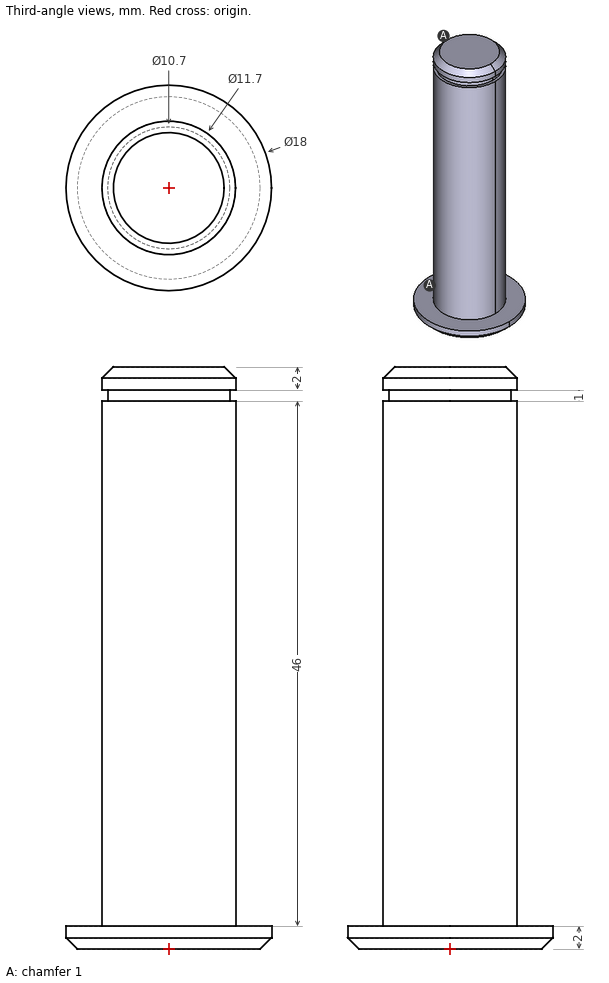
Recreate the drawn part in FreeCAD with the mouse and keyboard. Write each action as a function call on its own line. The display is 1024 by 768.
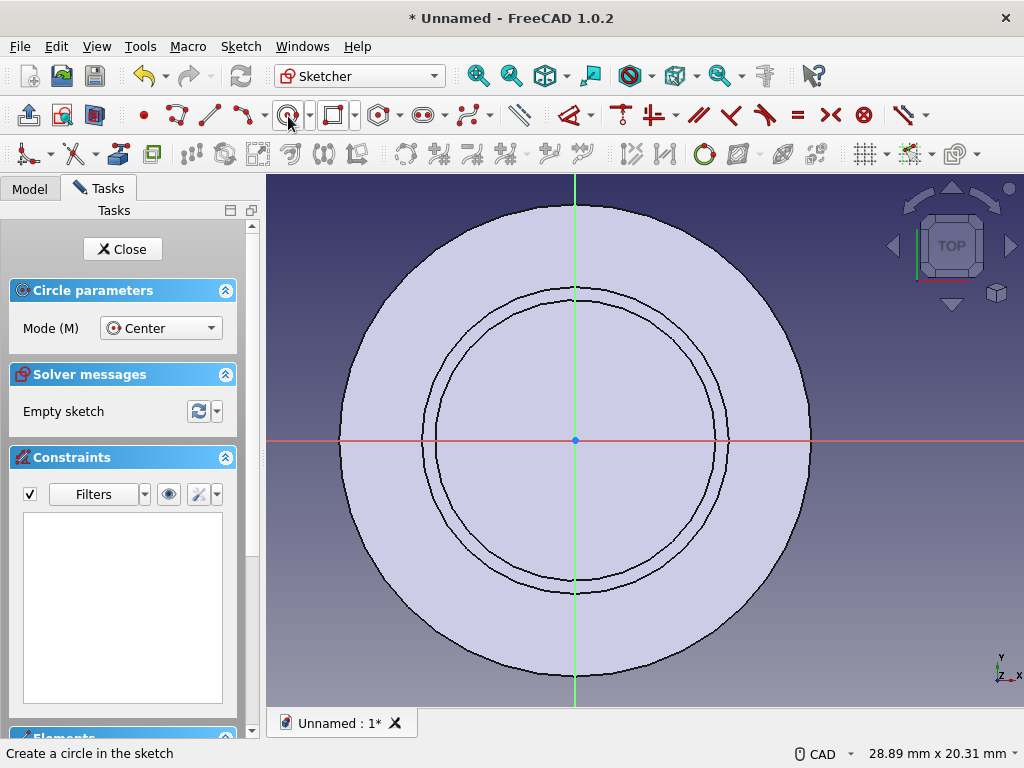
click(575, 440)
move(684, 332)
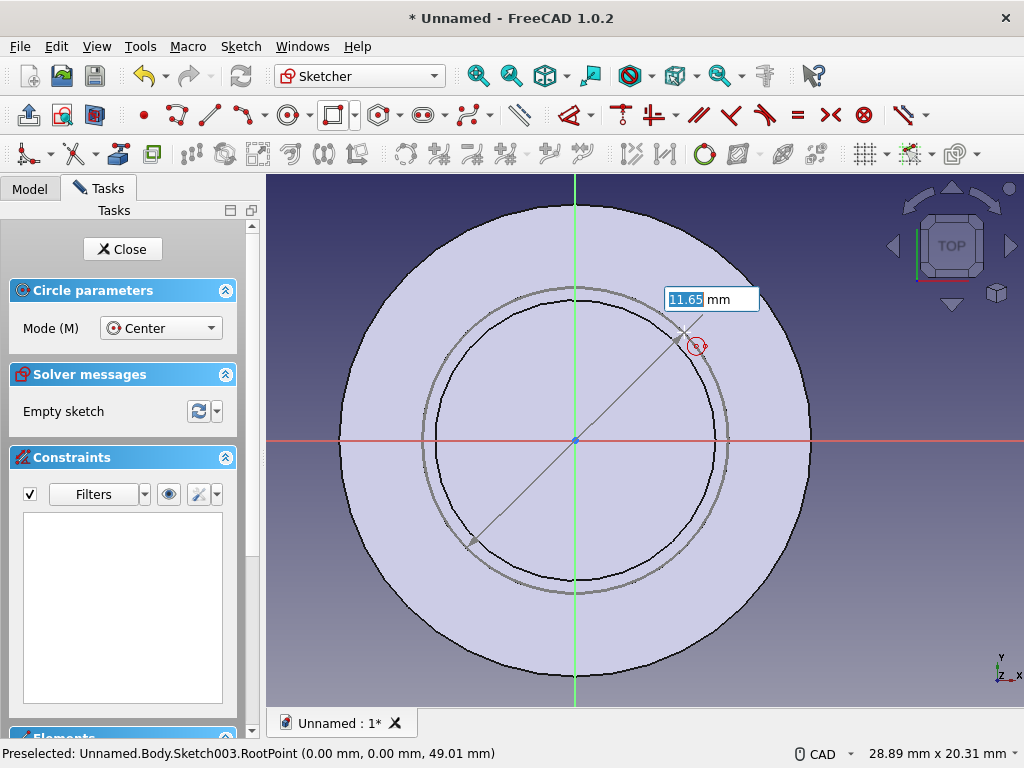
text(11.7)
key(Return)
key(Escape)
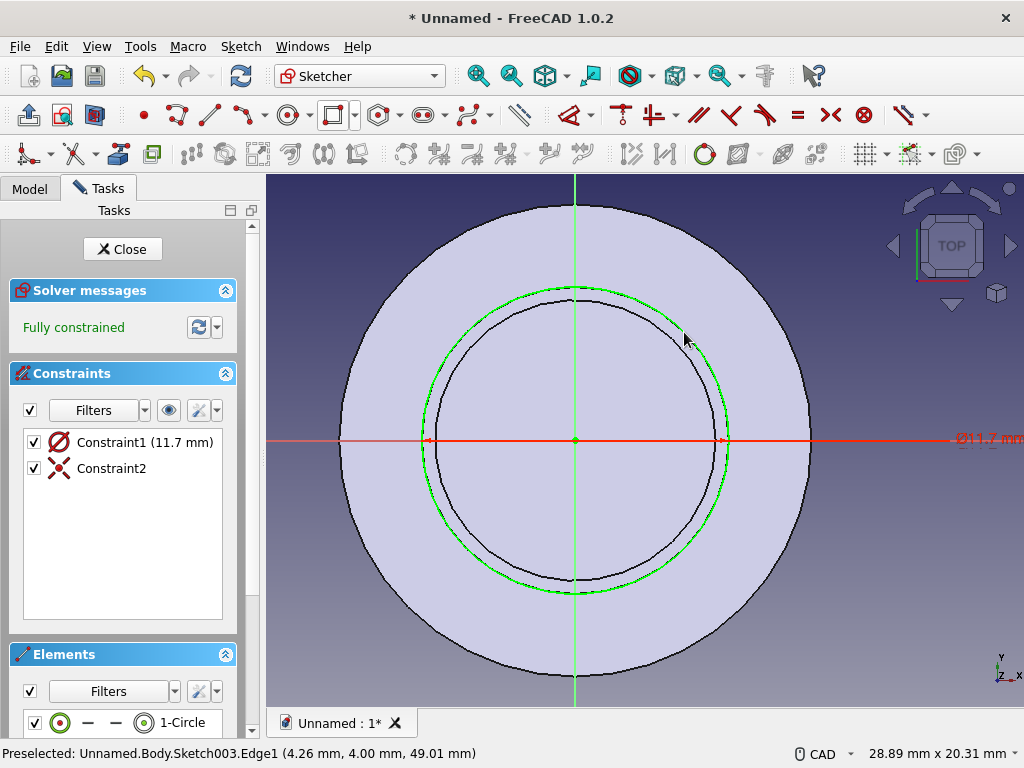
click(123, 249)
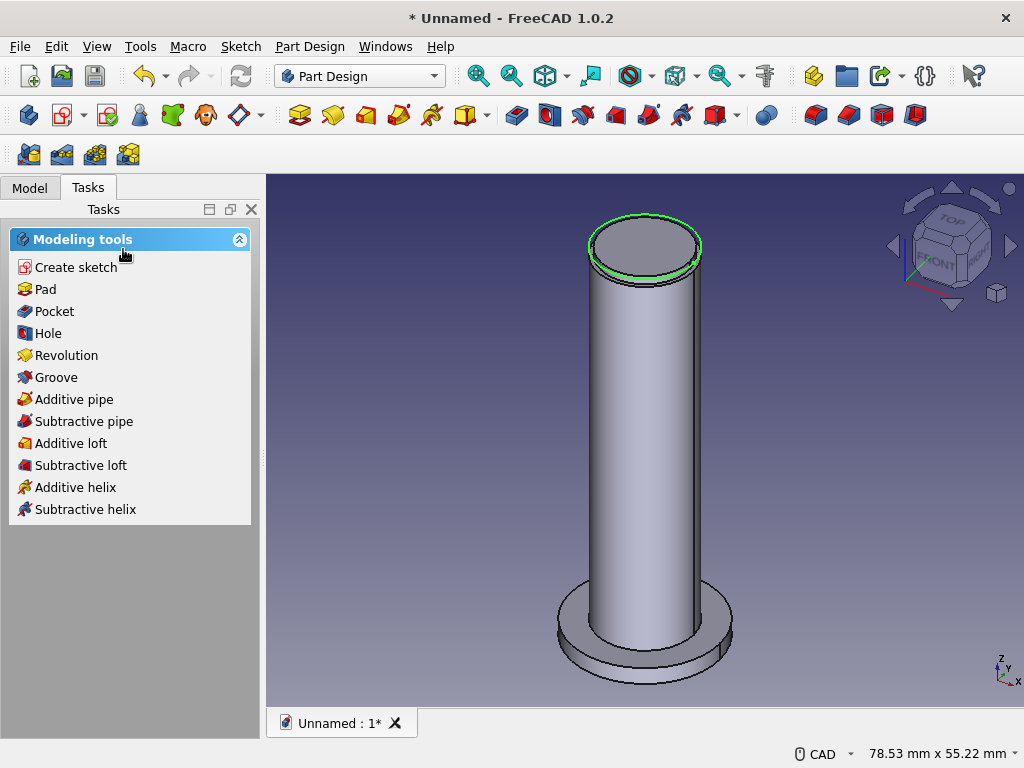
click(300, 116)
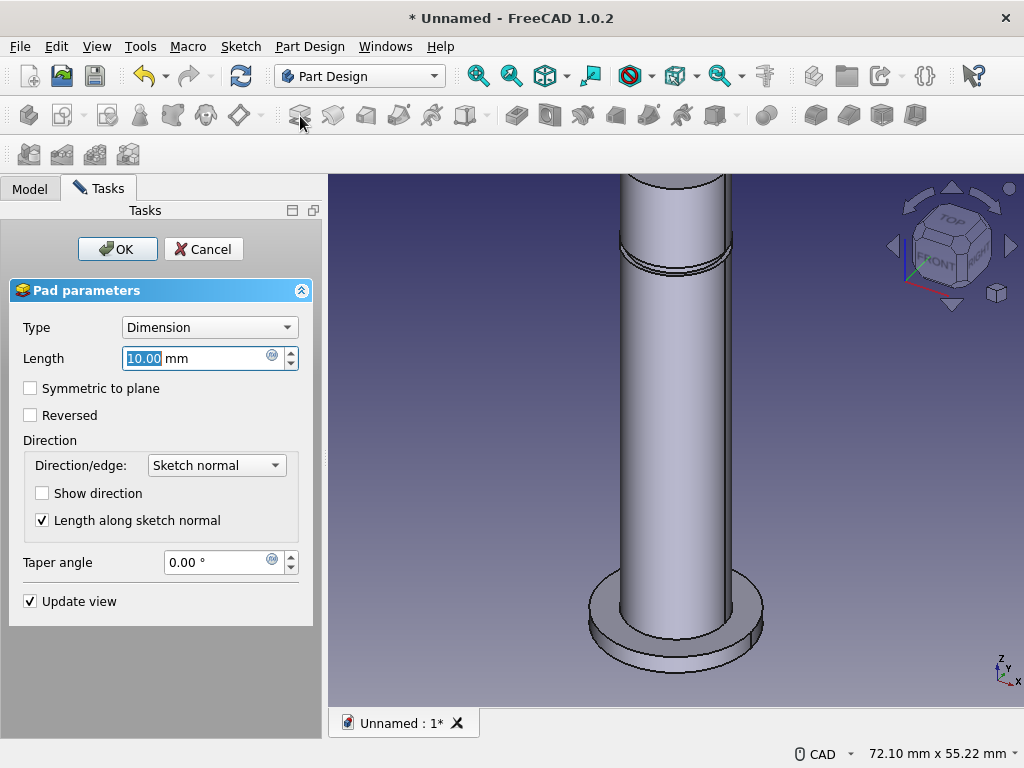
text(2)
key(Tab)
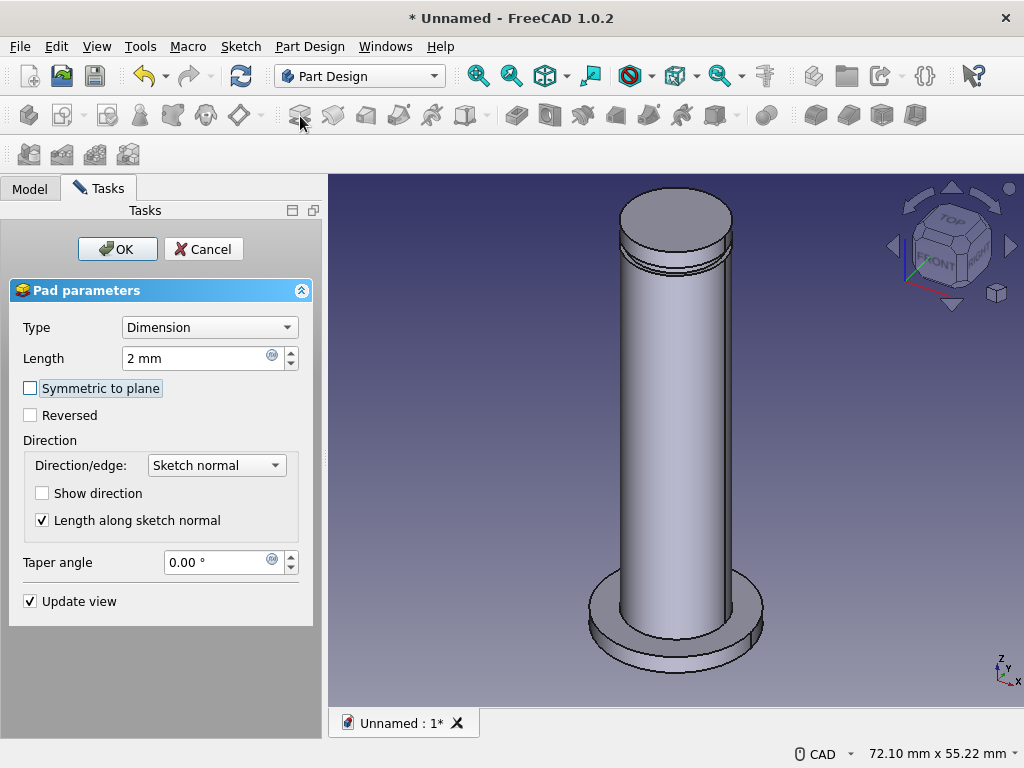
click(118, 249)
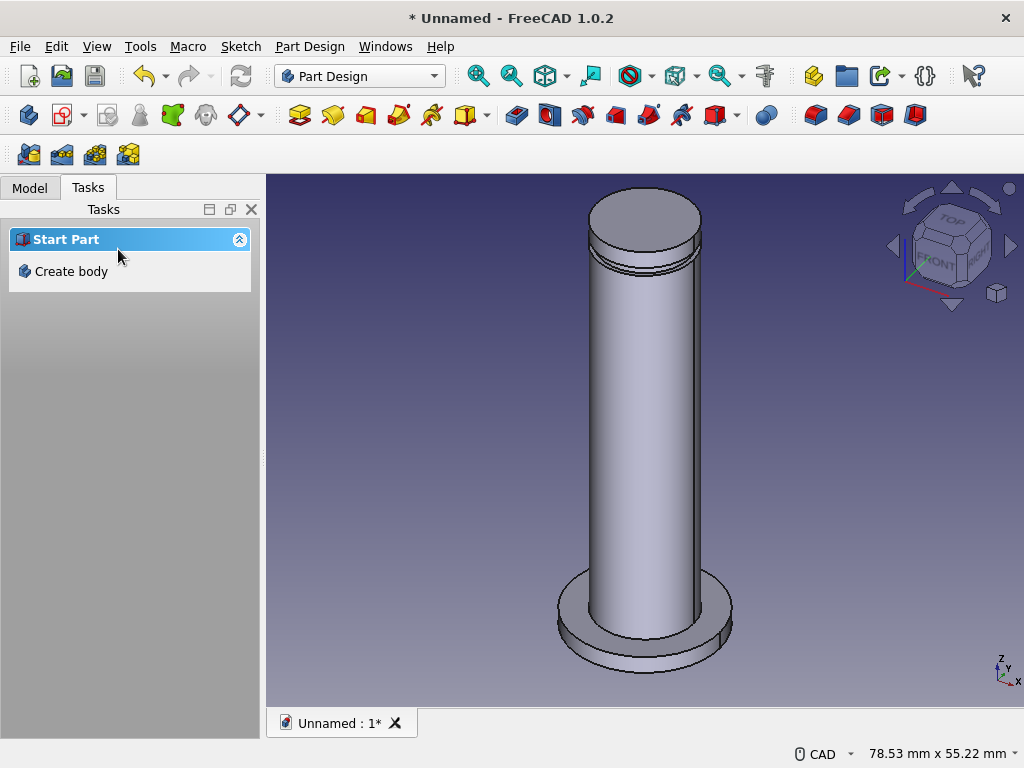
click(479, 76)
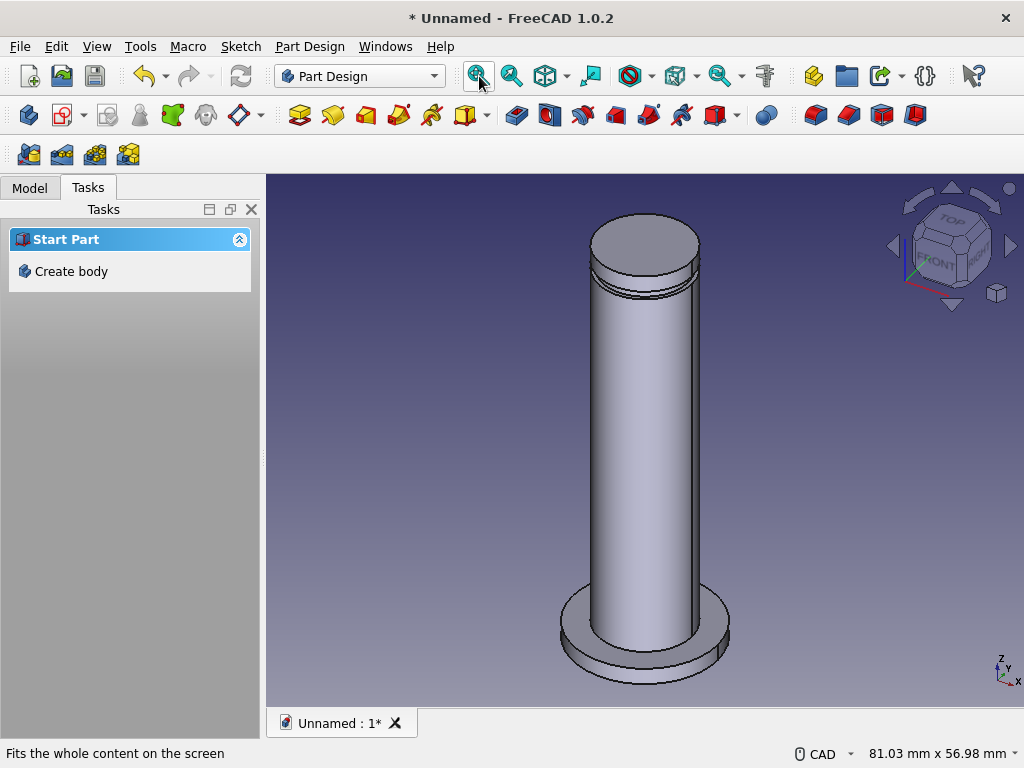
click(591, 247)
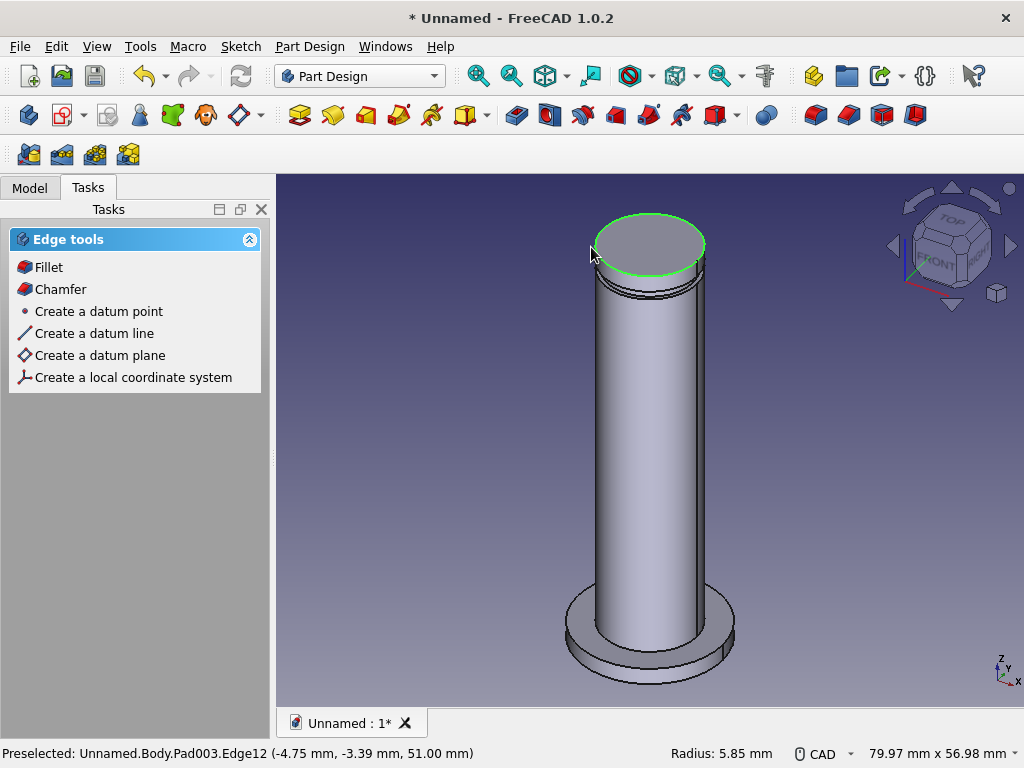
key(0)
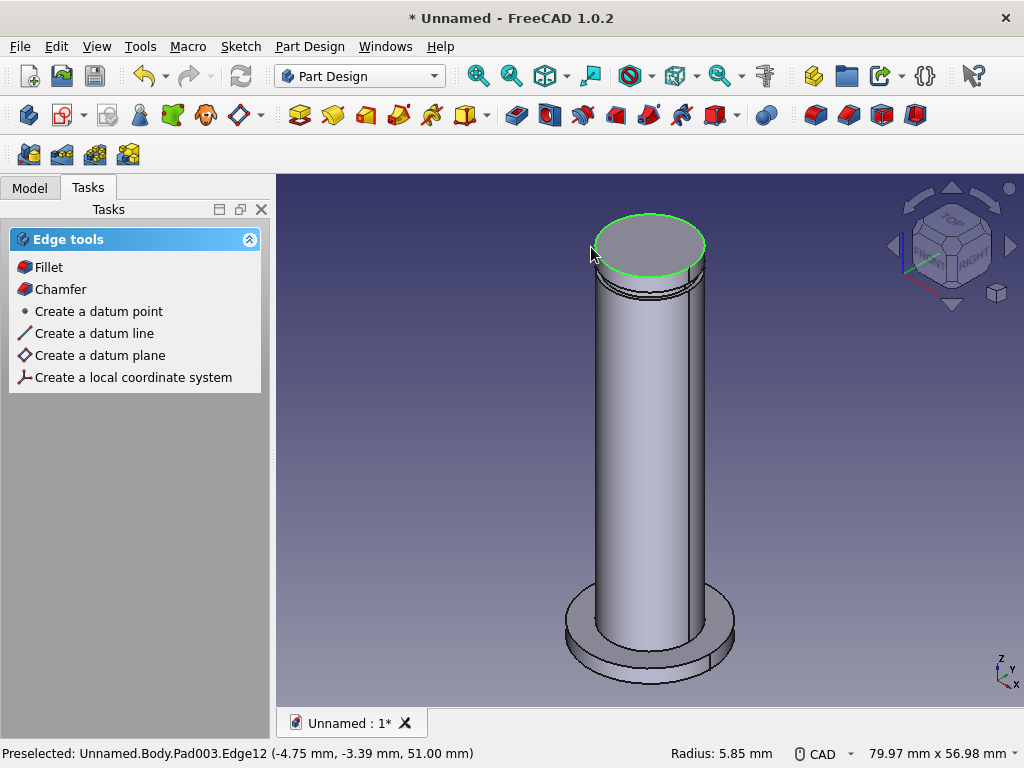
key(2)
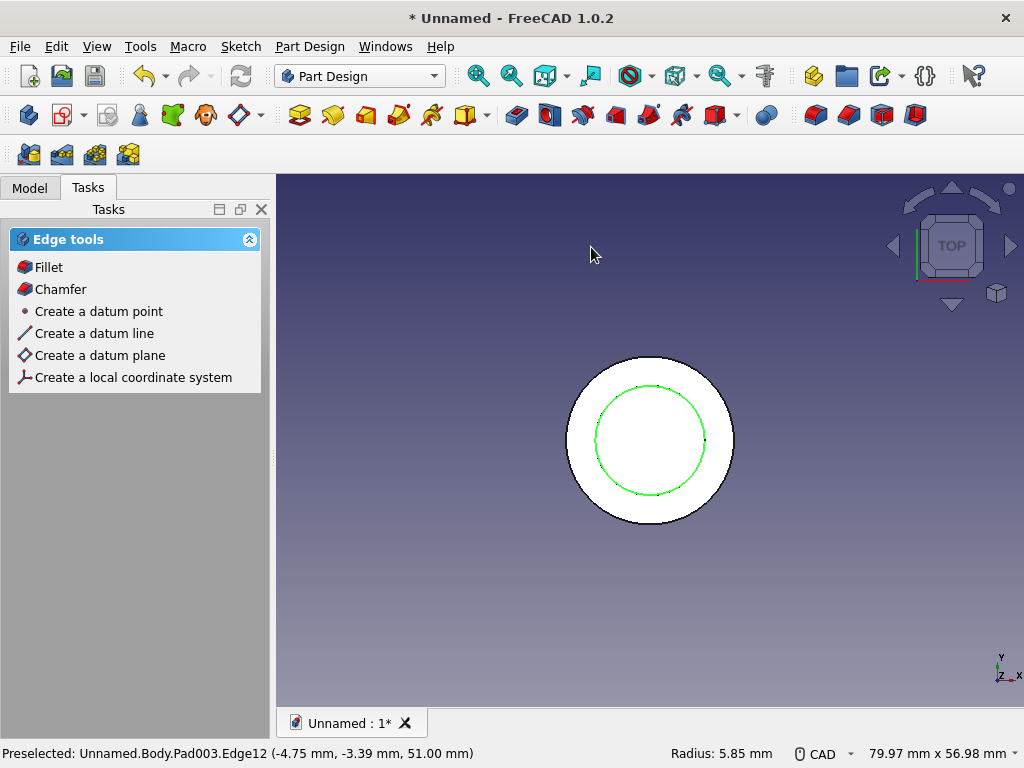
click(479, 76)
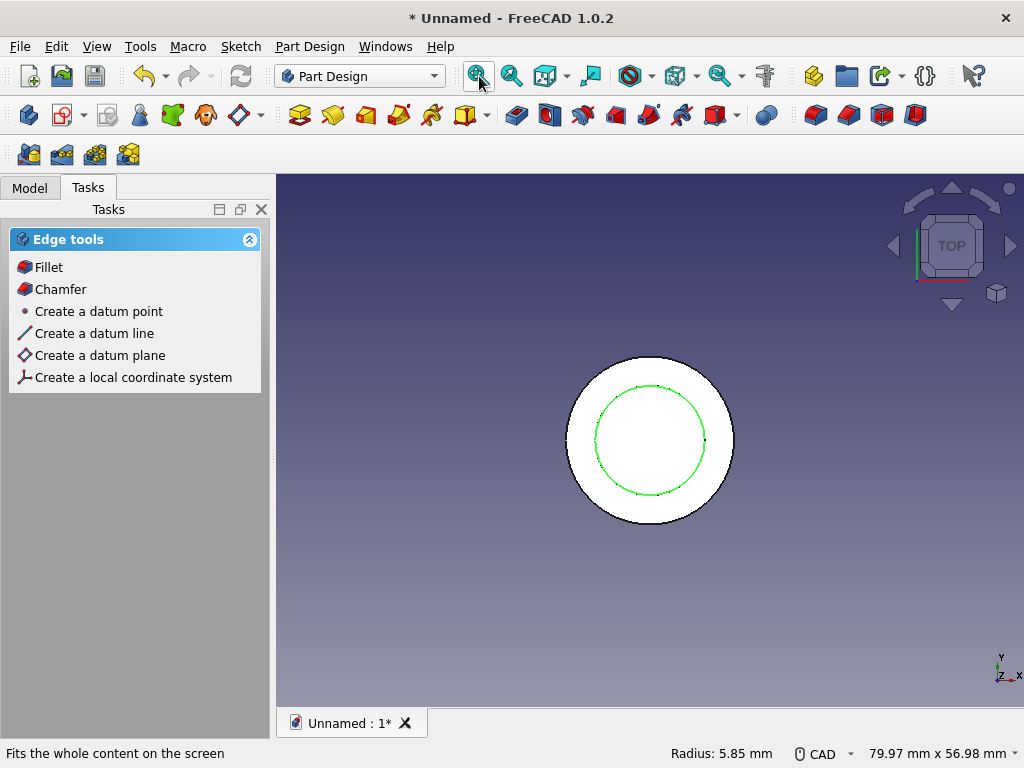
key(1)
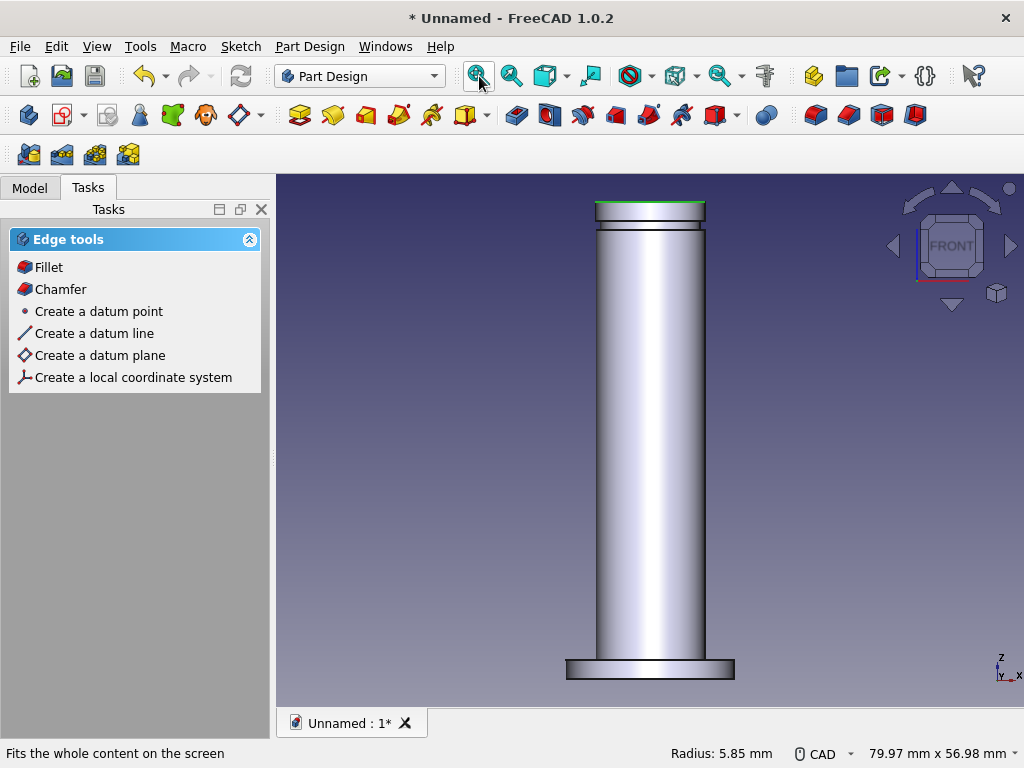
click(582, 678, ctrl)